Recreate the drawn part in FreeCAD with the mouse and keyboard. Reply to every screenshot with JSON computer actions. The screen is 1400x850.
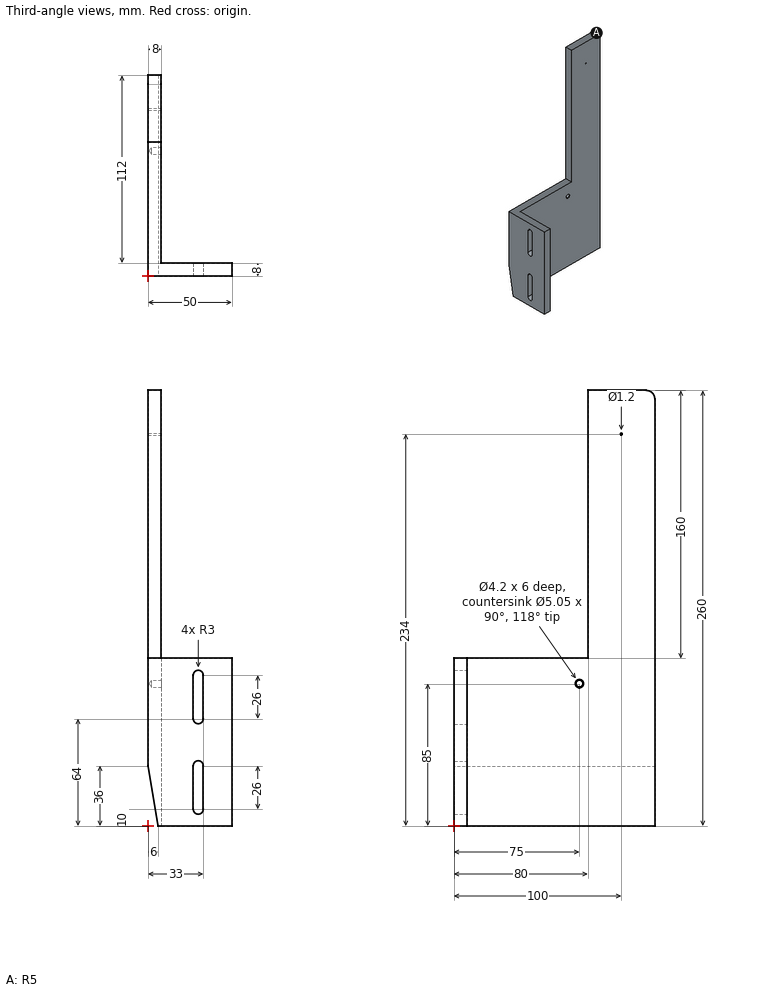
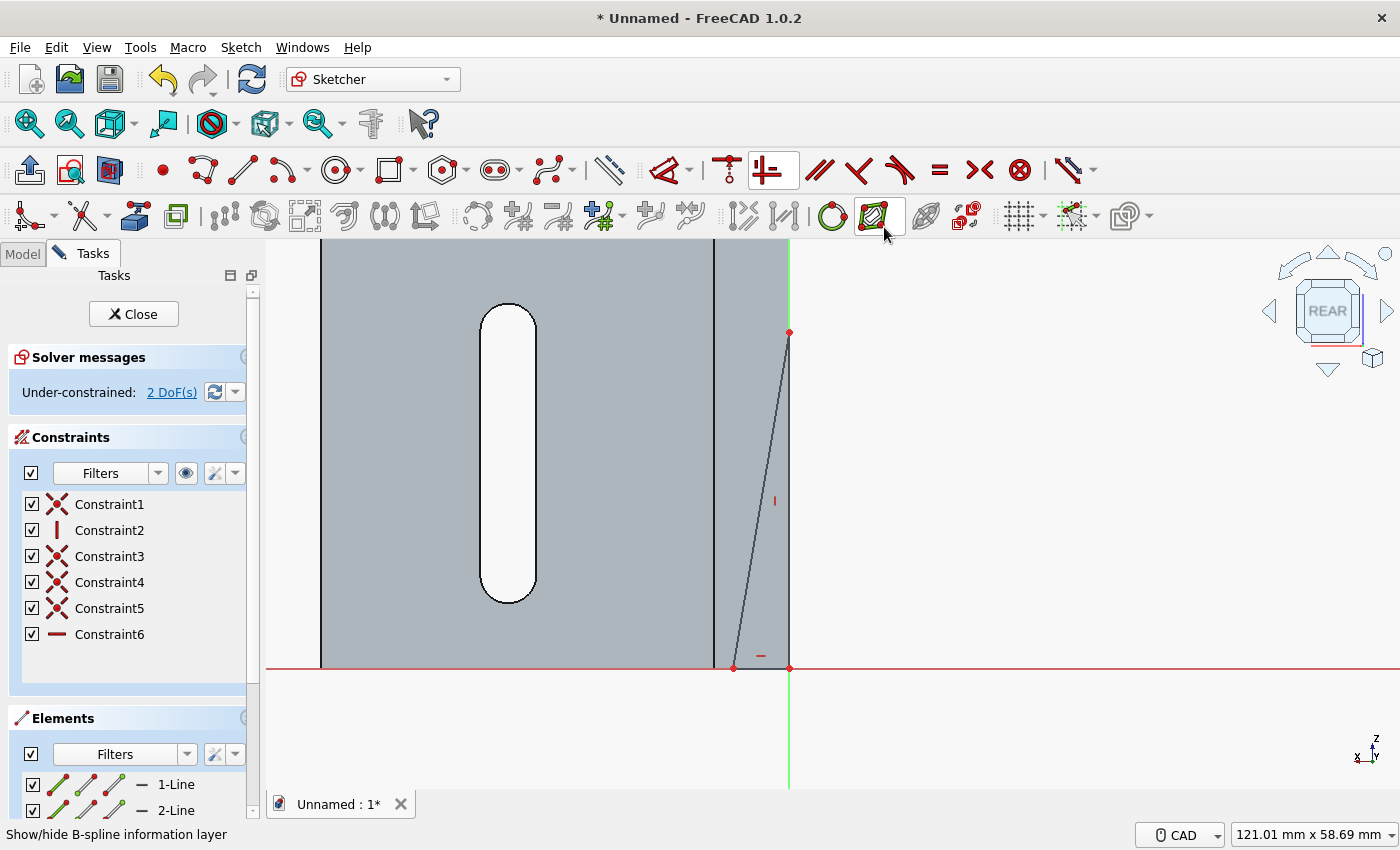
{"action": "left_click", "coordinate": [664, 170]}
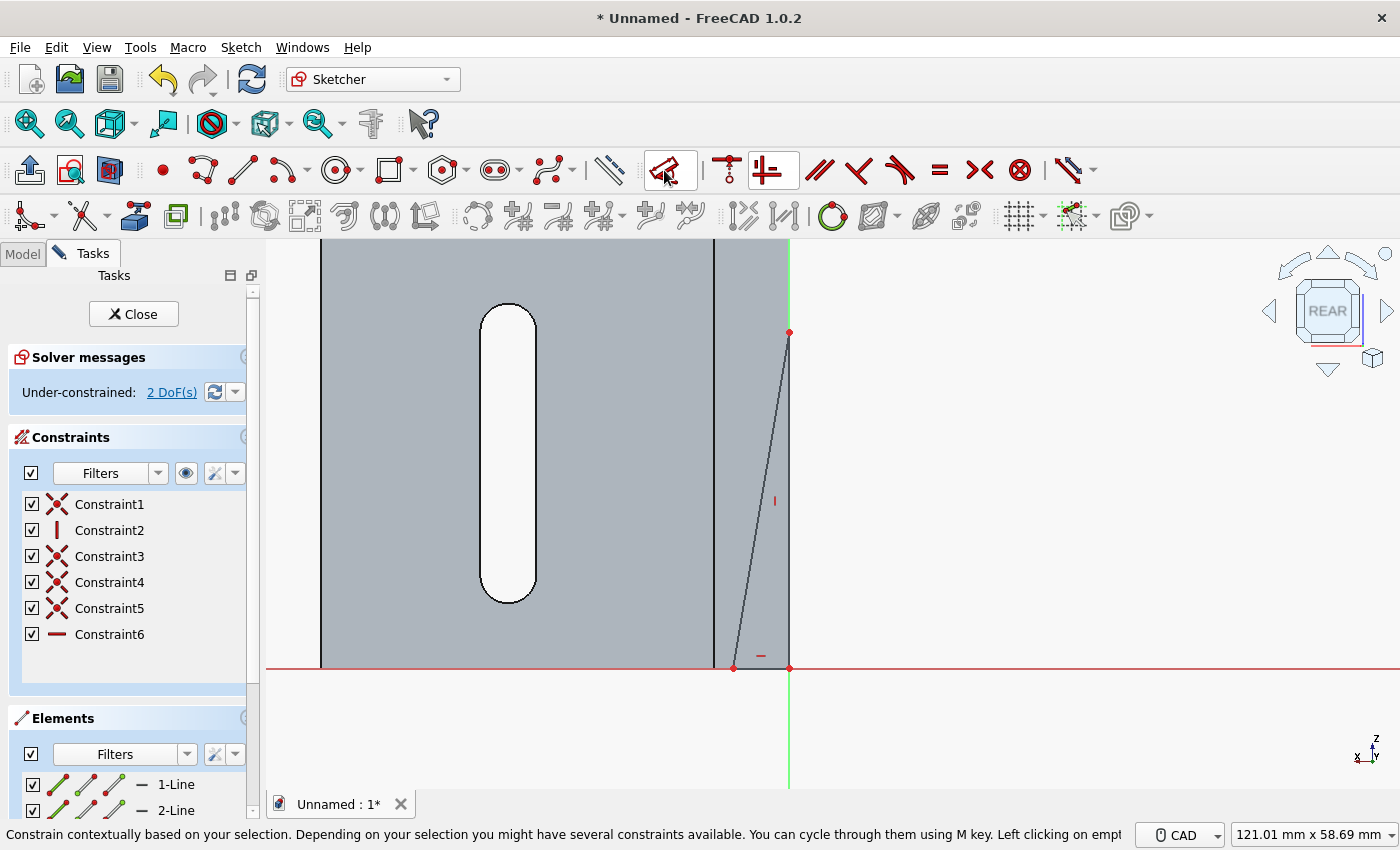
{"action": "left_click", "coordinate": [750, 669]}
{"action": "left_click", "coordinate": [761, 703]}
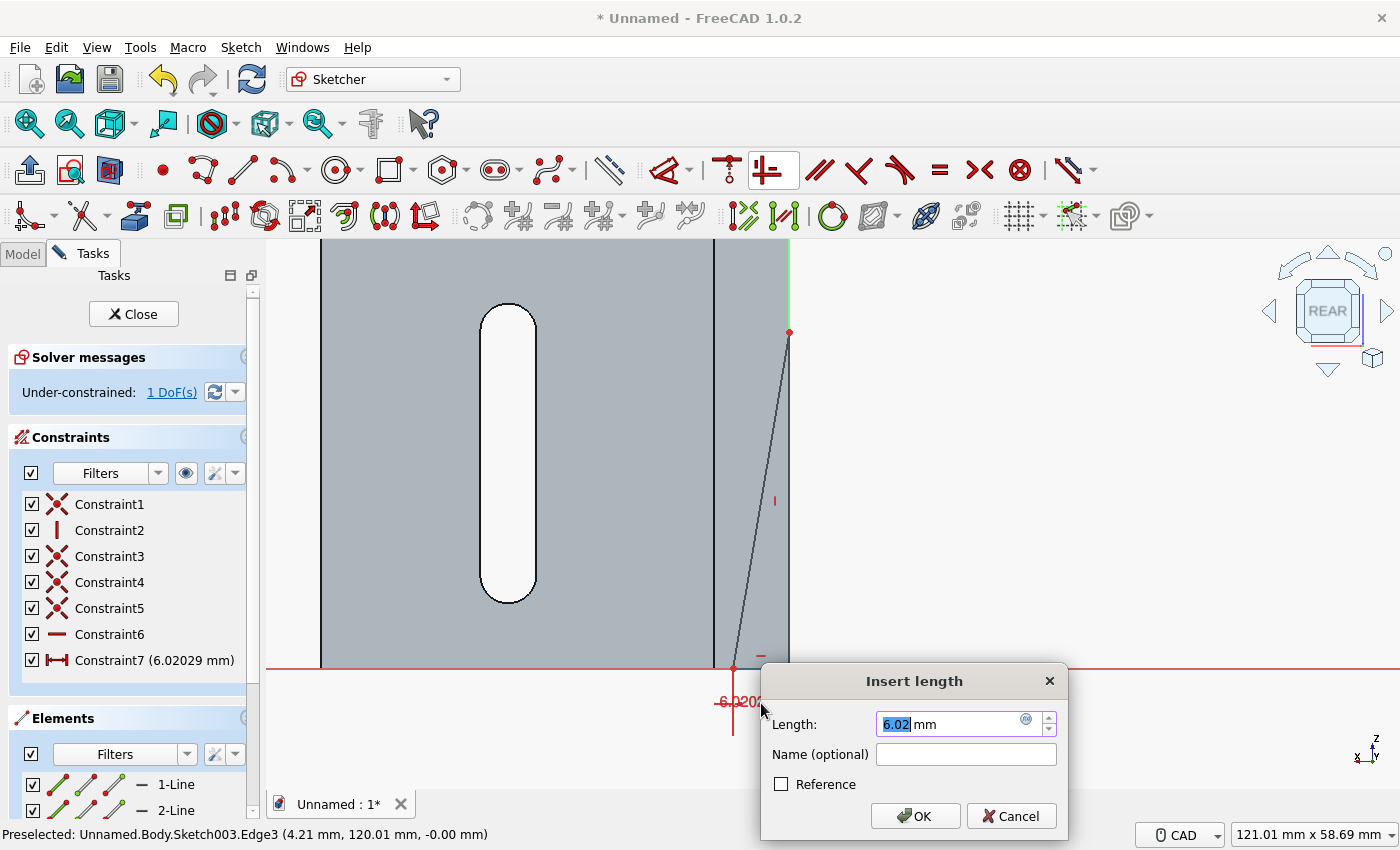
{"action": "type", "text": "6"}
{"action": "key", "text": "Return"}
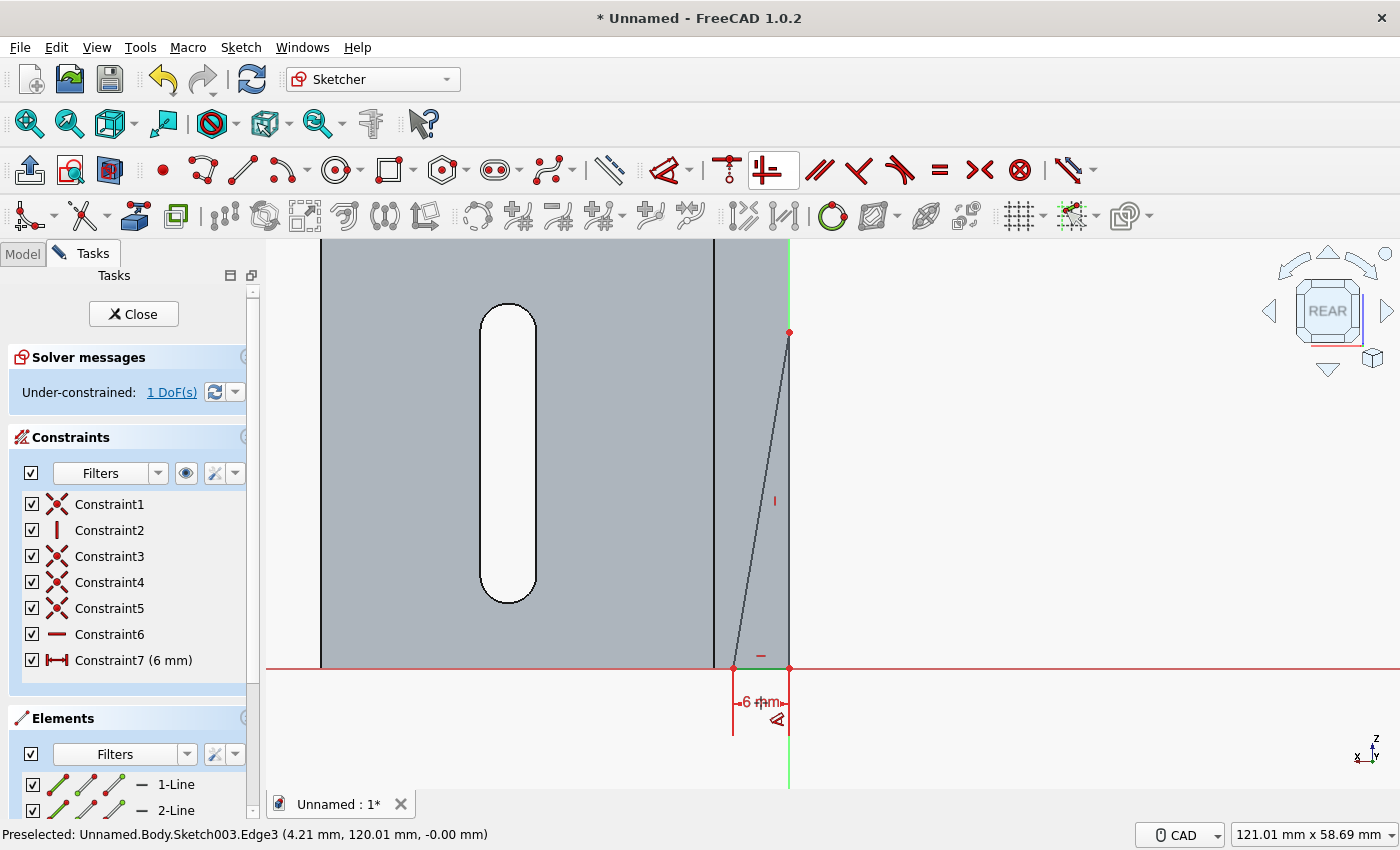
{"action": "left_click", "coordinate": [789, 568]}
{"action": "left_click", "coordinate": [823, 501]}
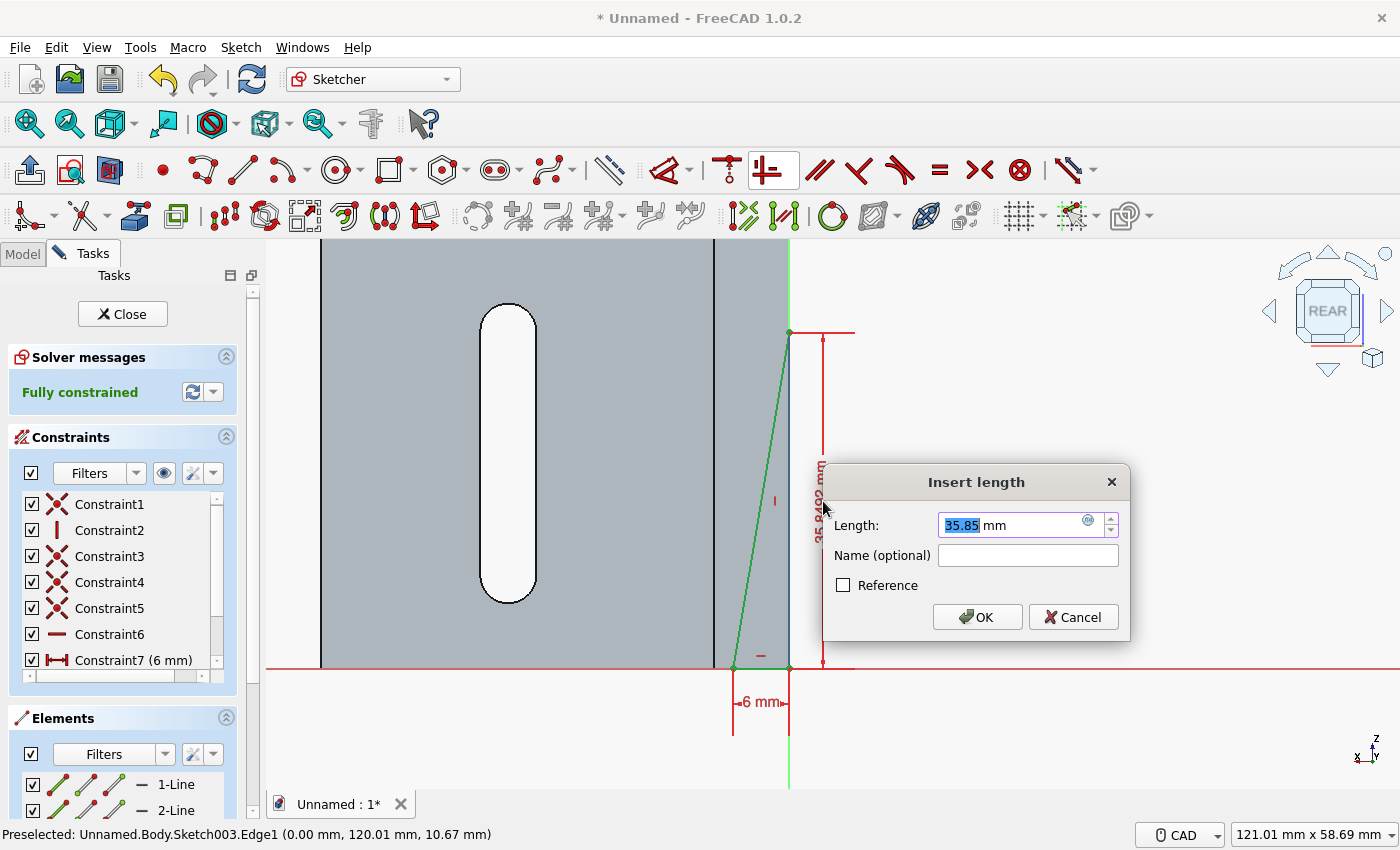
{"action": "type", "text": "36"}
{"action": "key", "text": "Return"}
{"action": "key", "text": "Escape"}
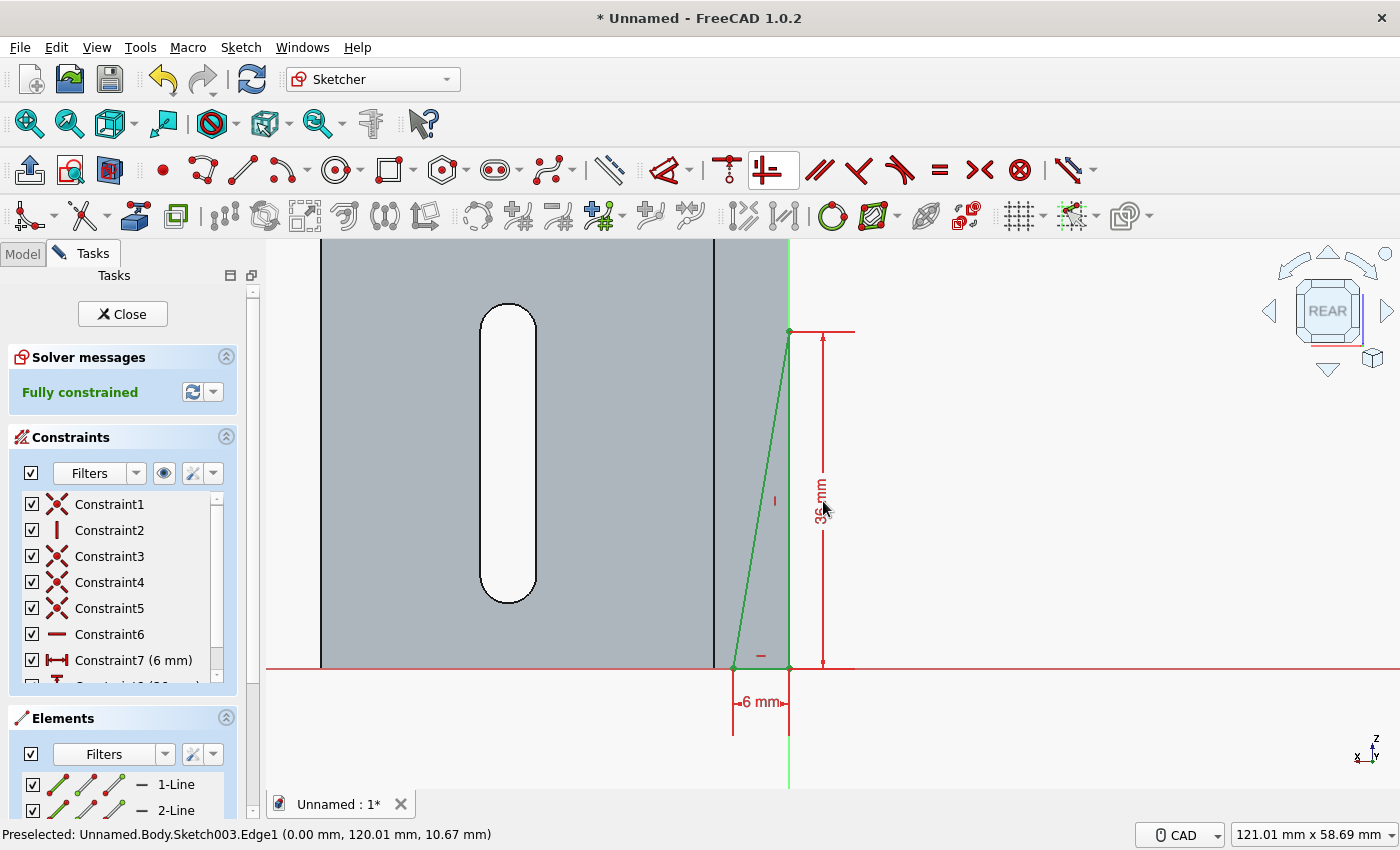
{"action": "left_click", "coordinate": [123, 314]}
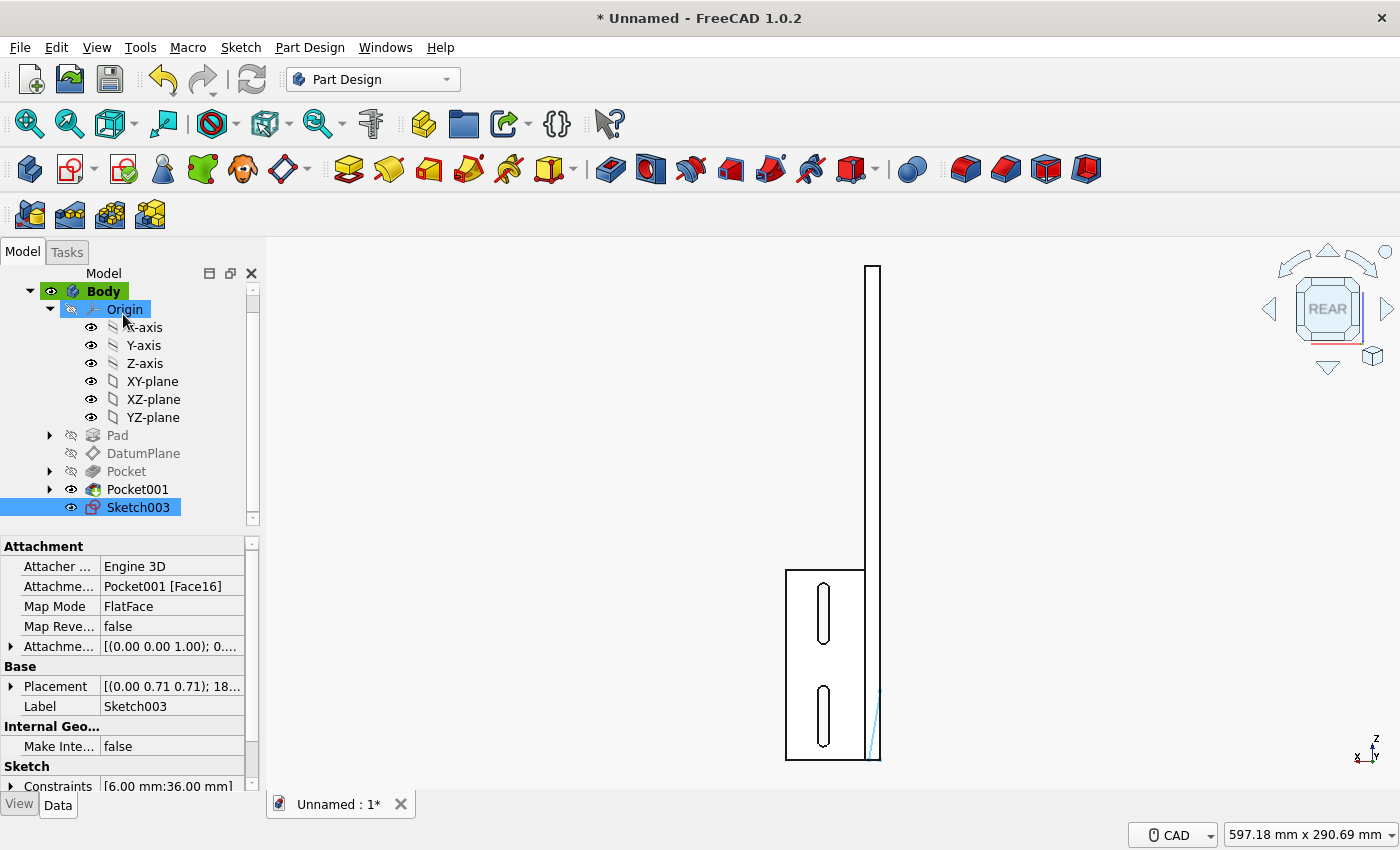
{"action": "left_click", "coordinate": [612, 170]}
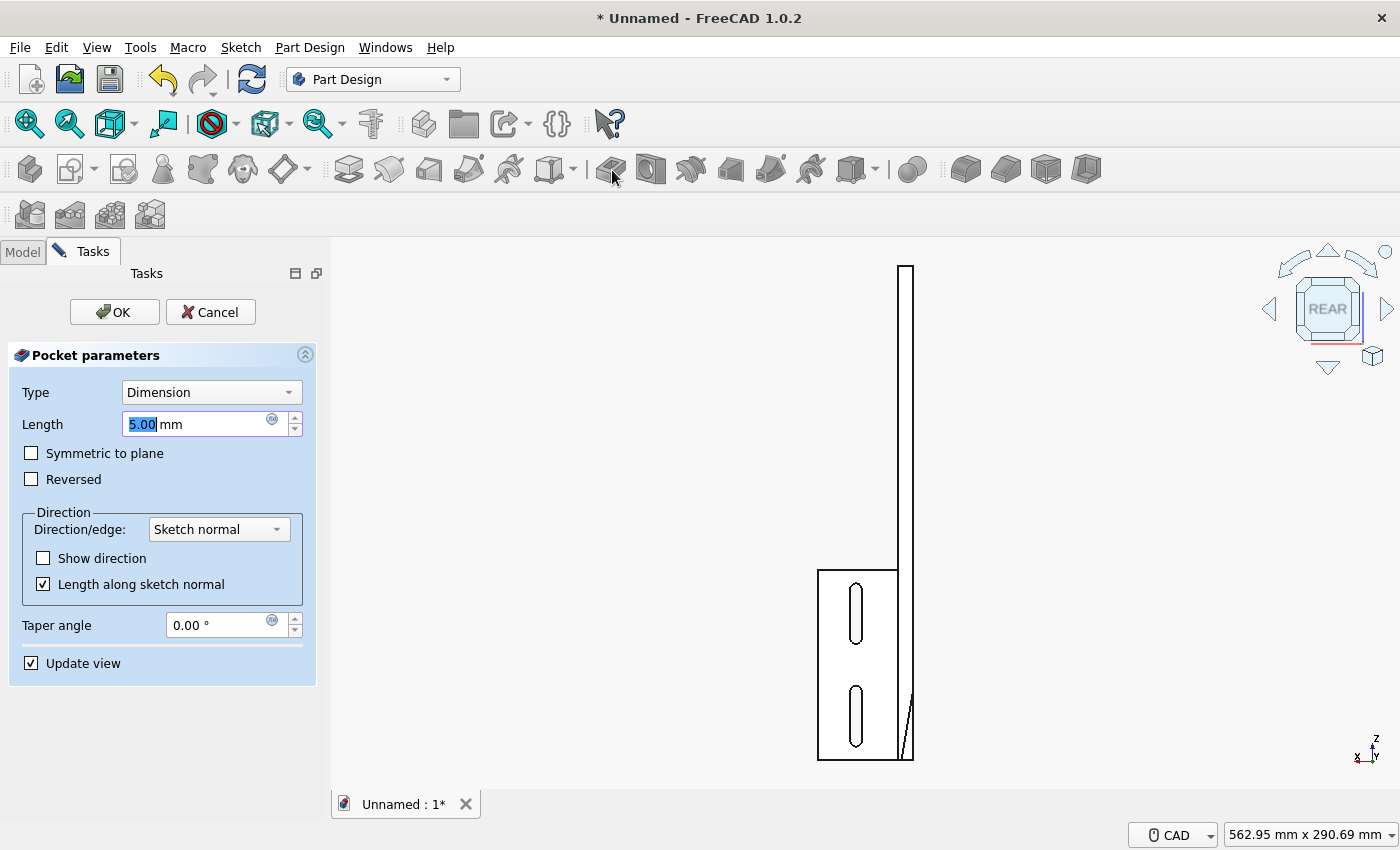
{"action": "left_click", "coordinate": [212, 392]}